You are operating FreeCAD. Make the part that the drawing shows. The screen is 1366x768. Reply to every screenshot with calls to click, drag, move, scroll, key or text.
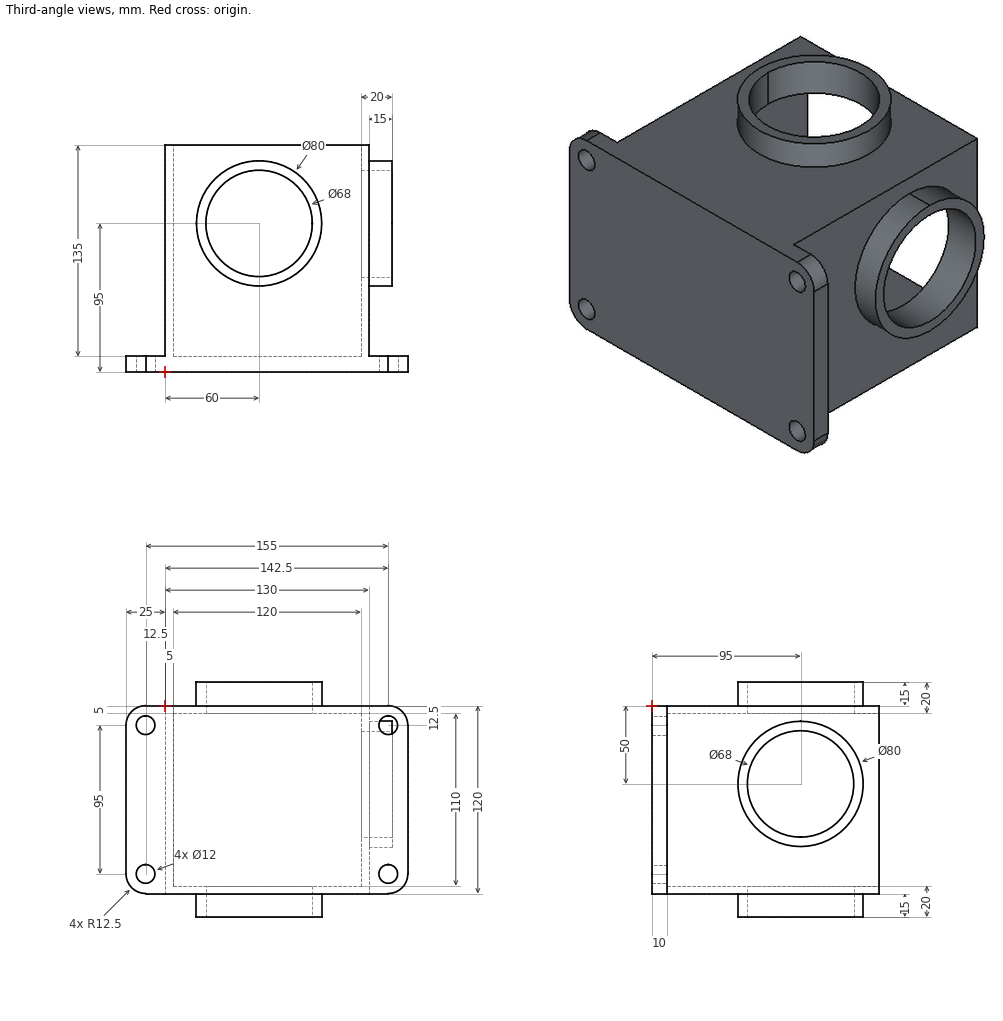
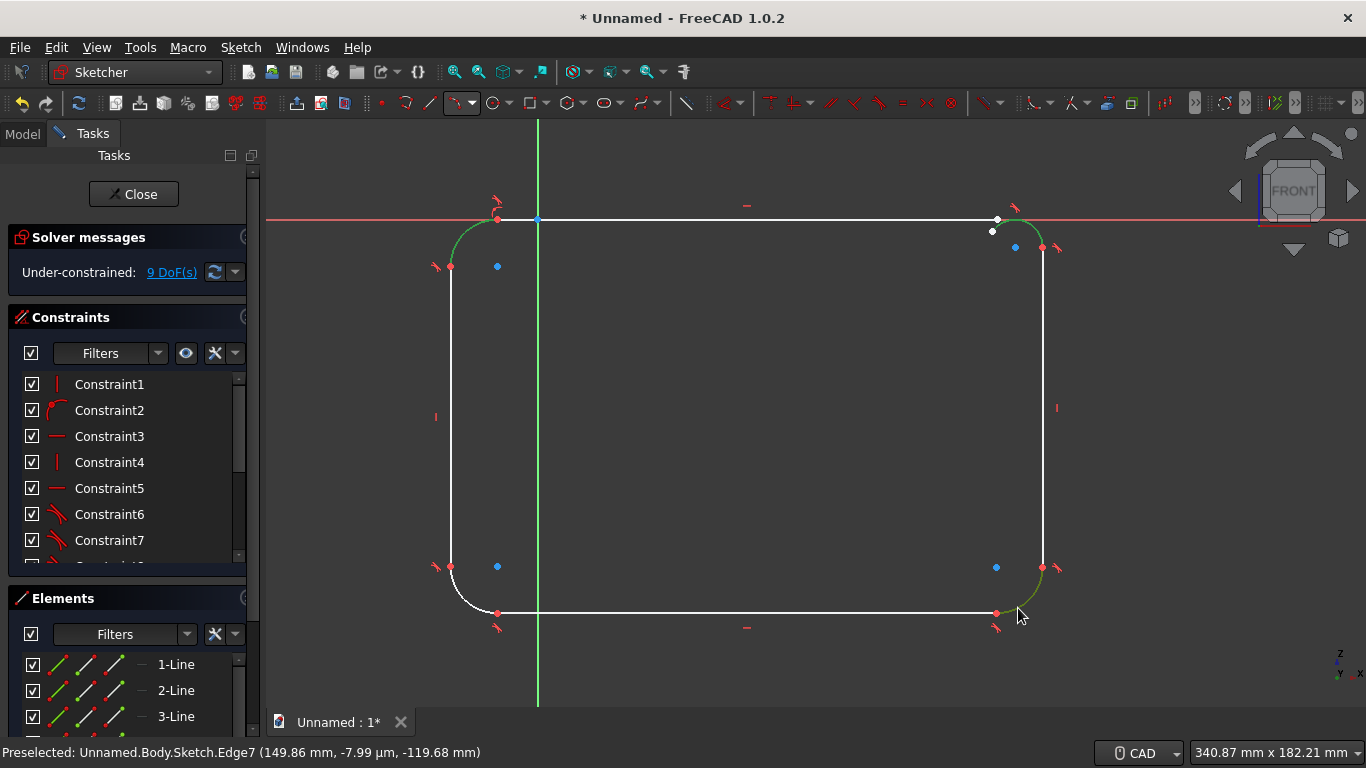
click(456, 588)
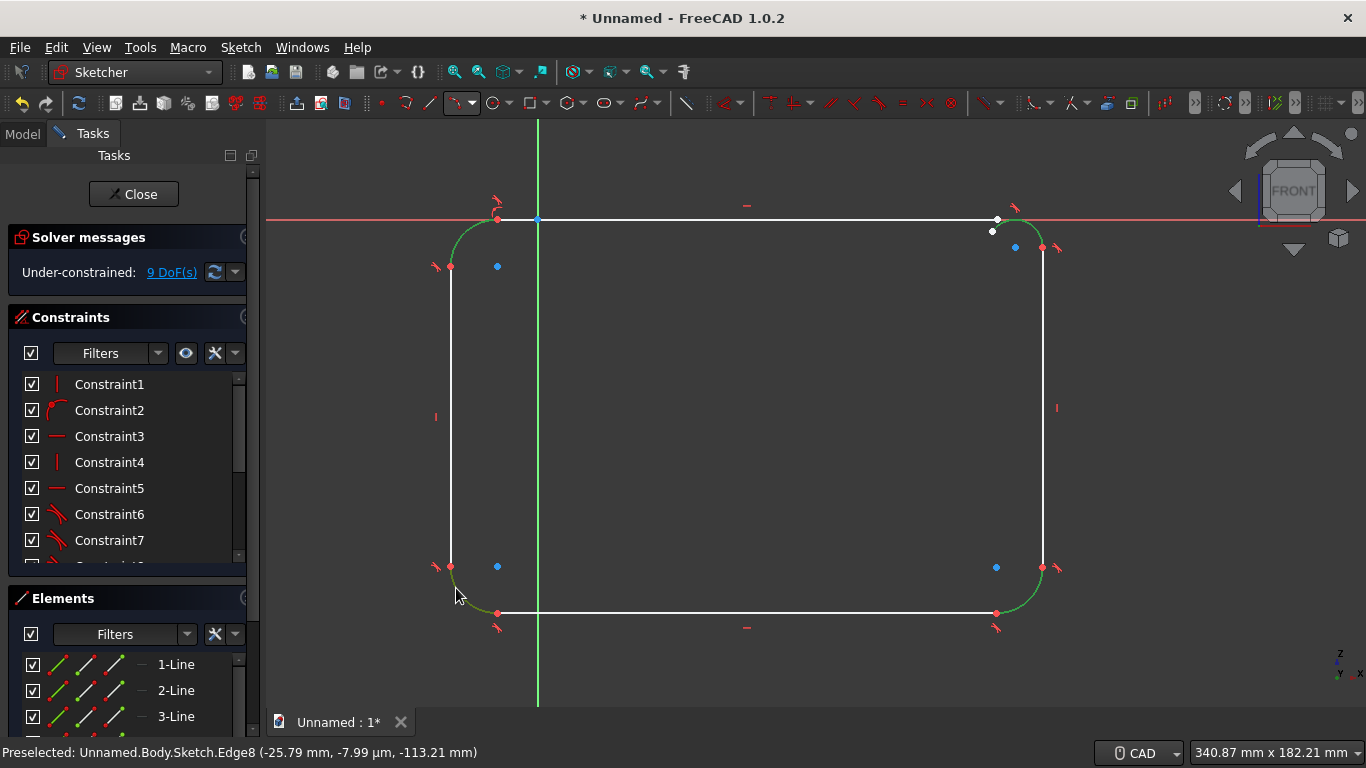
click(904, 104)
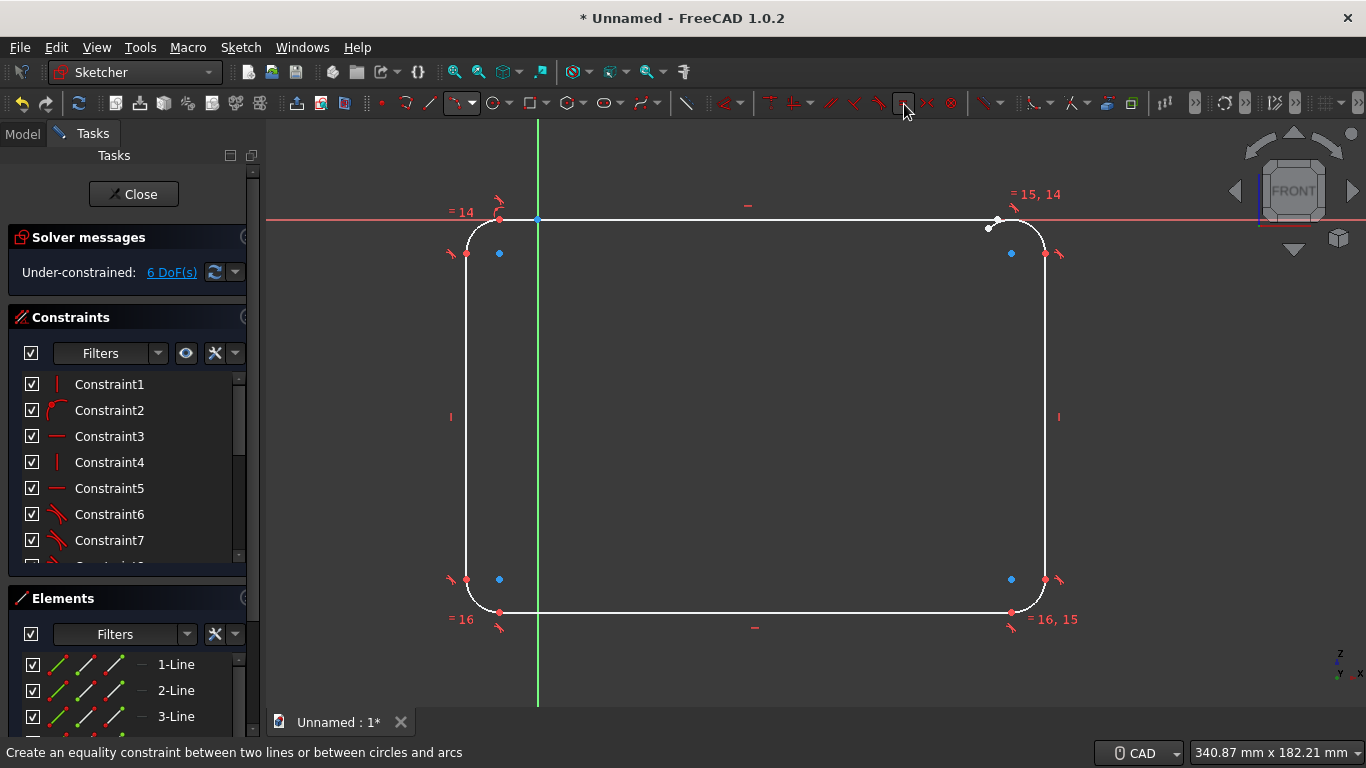
click(485, 223)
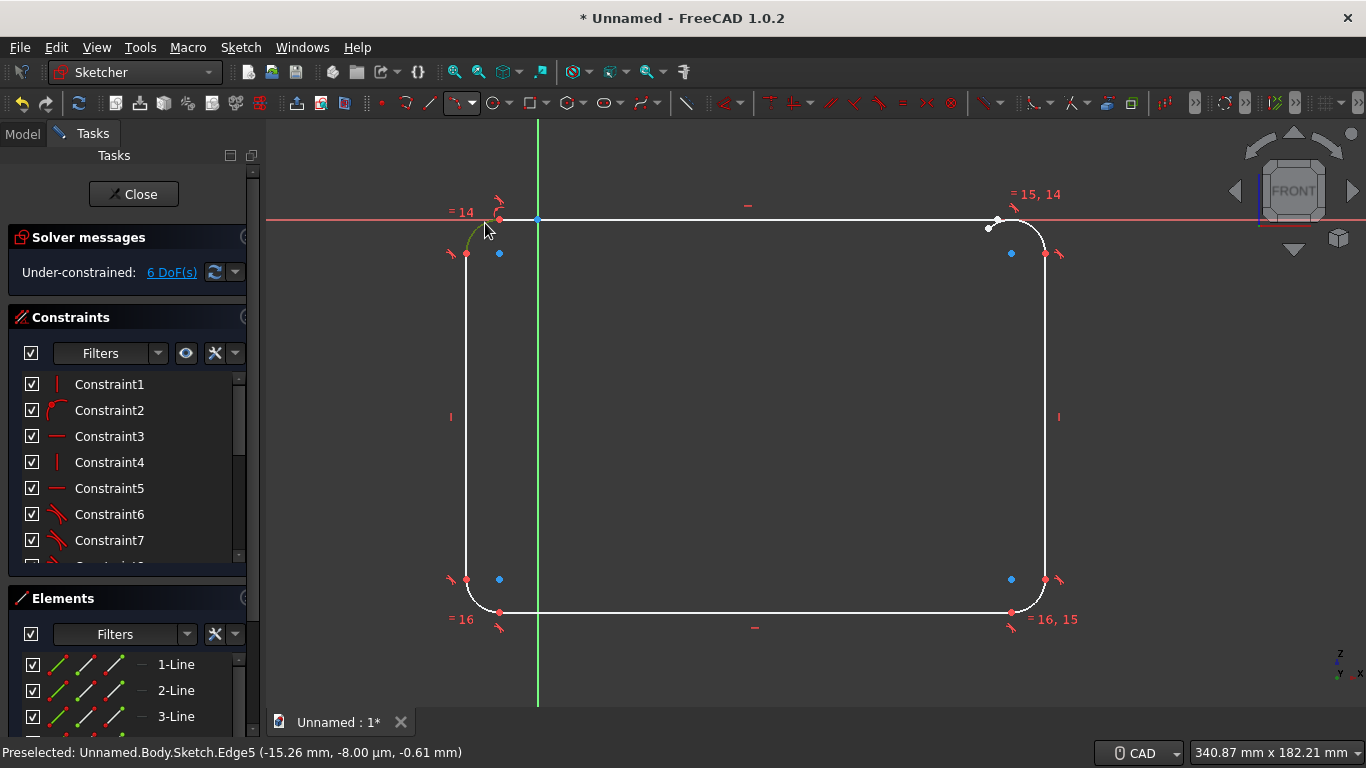
key(k)
key(r)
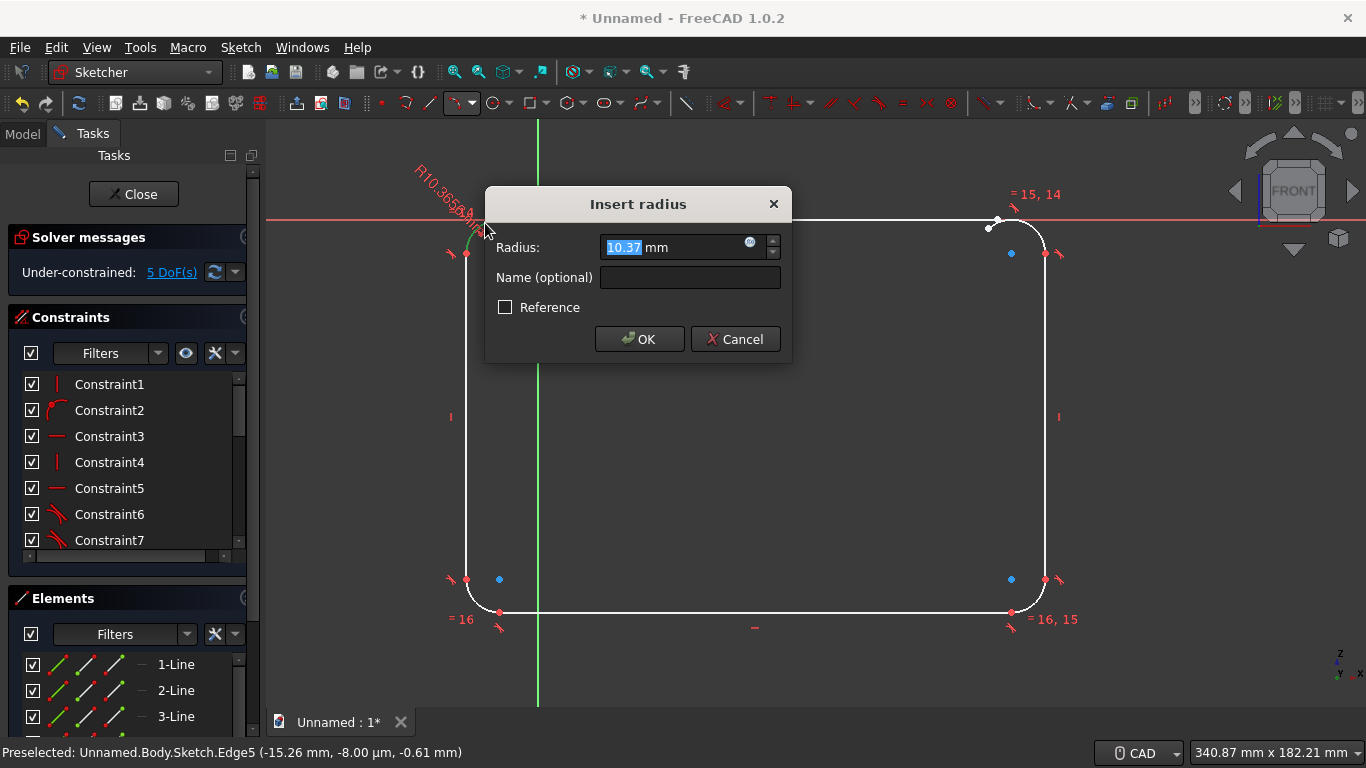
text(12.5)
key(Return)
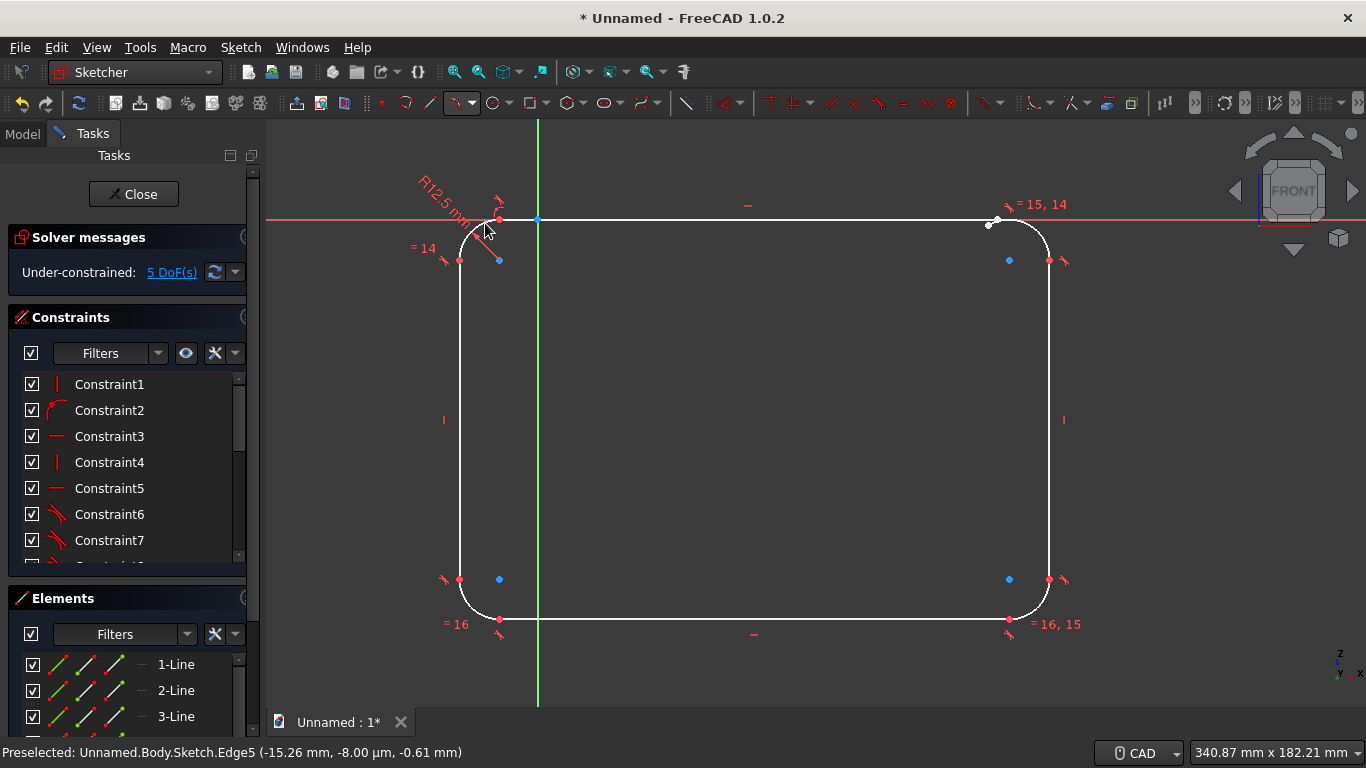
click(460, 483)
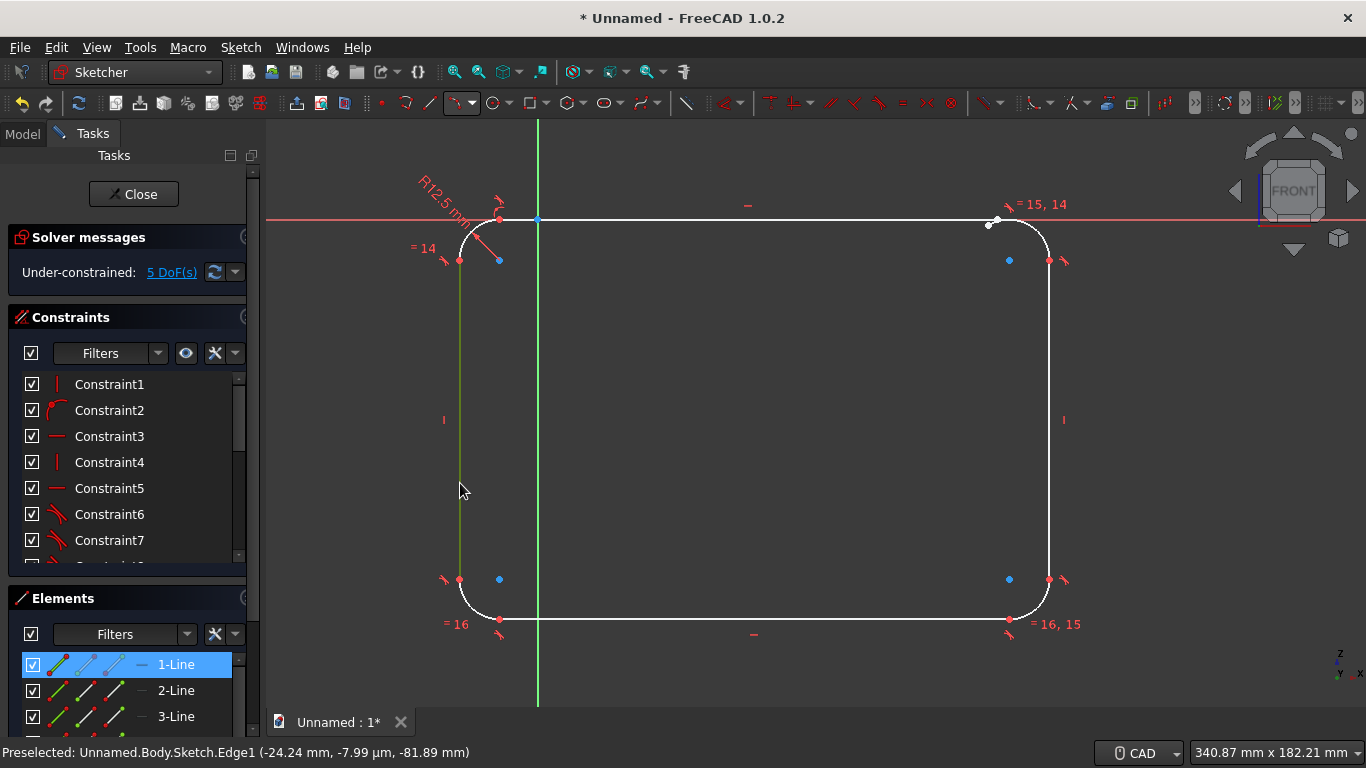
key(i)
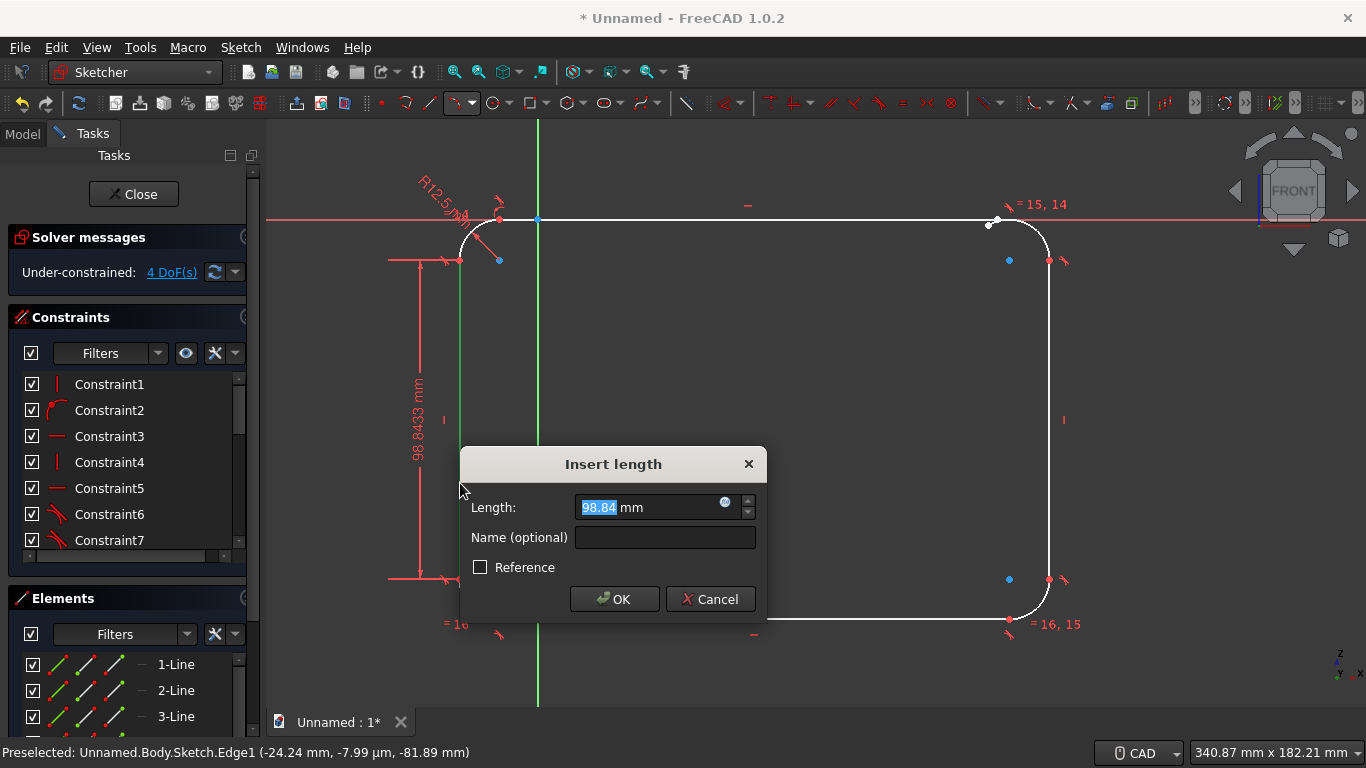
text(95)
key(Return)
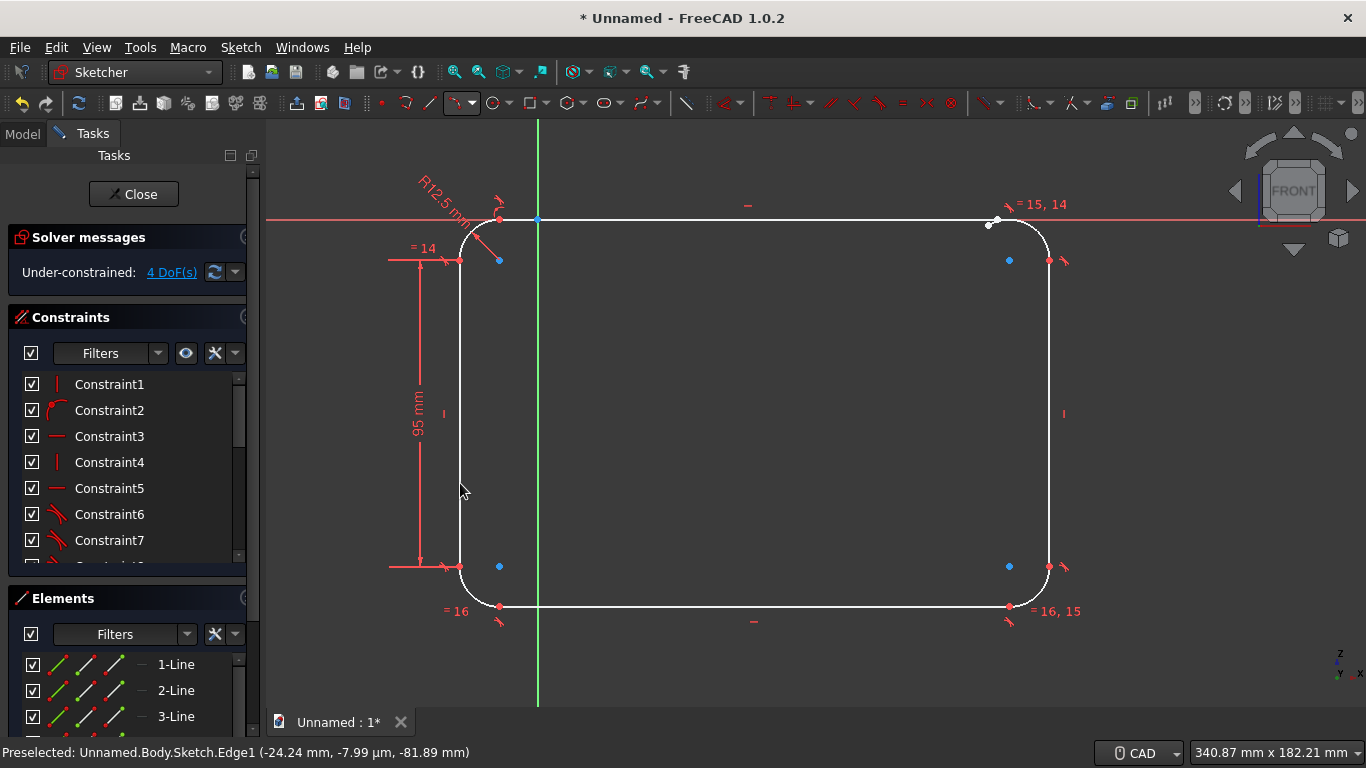
click(649, 220)